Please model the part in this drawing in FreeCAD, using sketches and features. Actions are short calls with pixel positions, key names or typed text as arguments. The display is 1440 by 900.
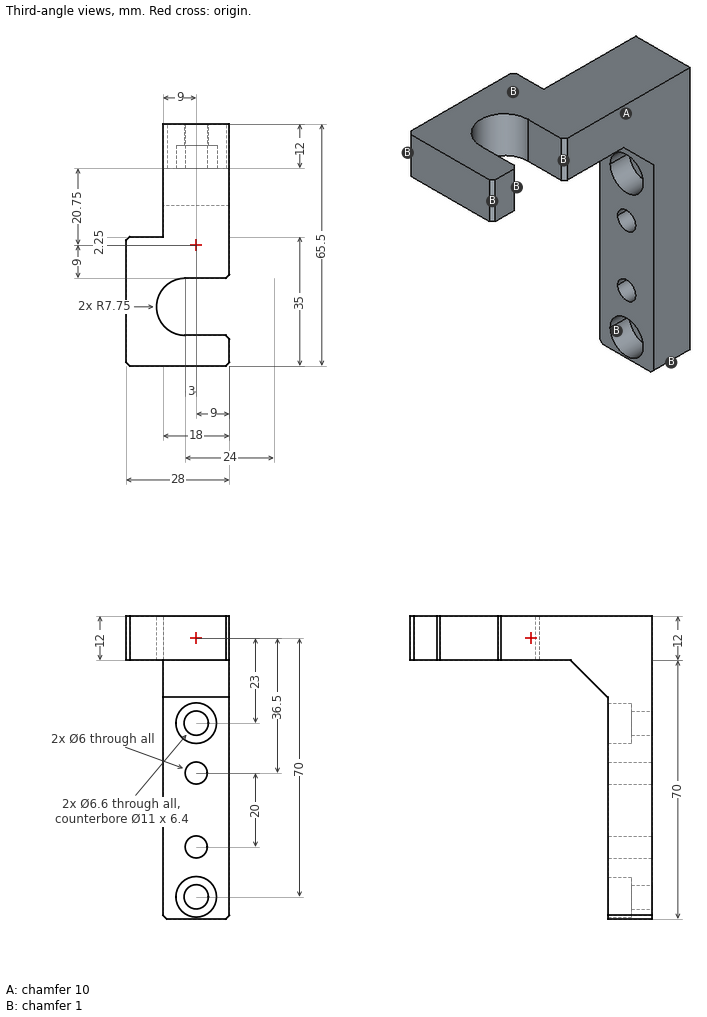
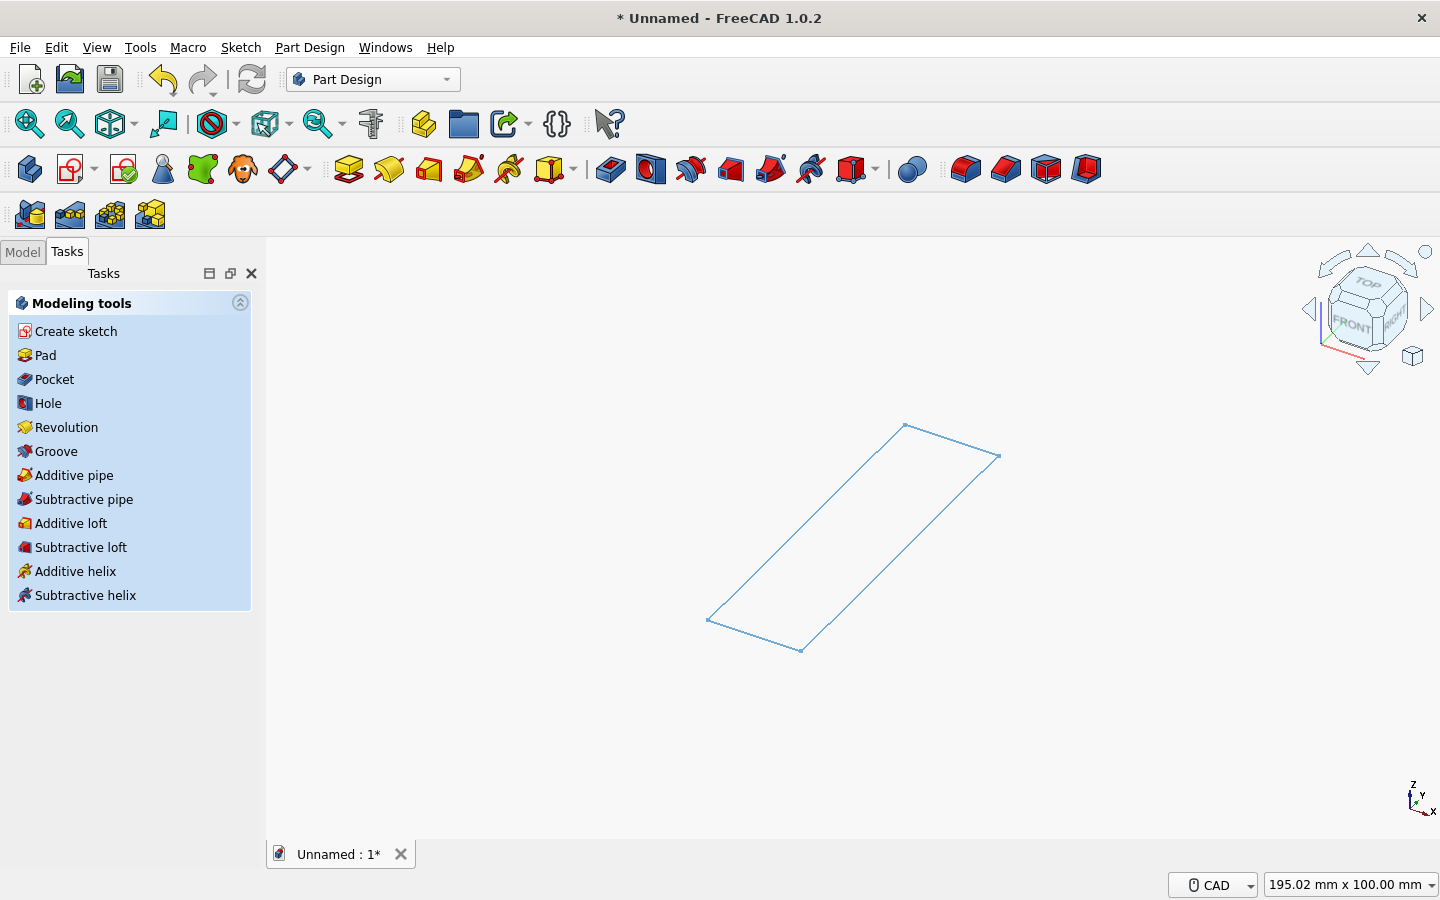
click(350, 170)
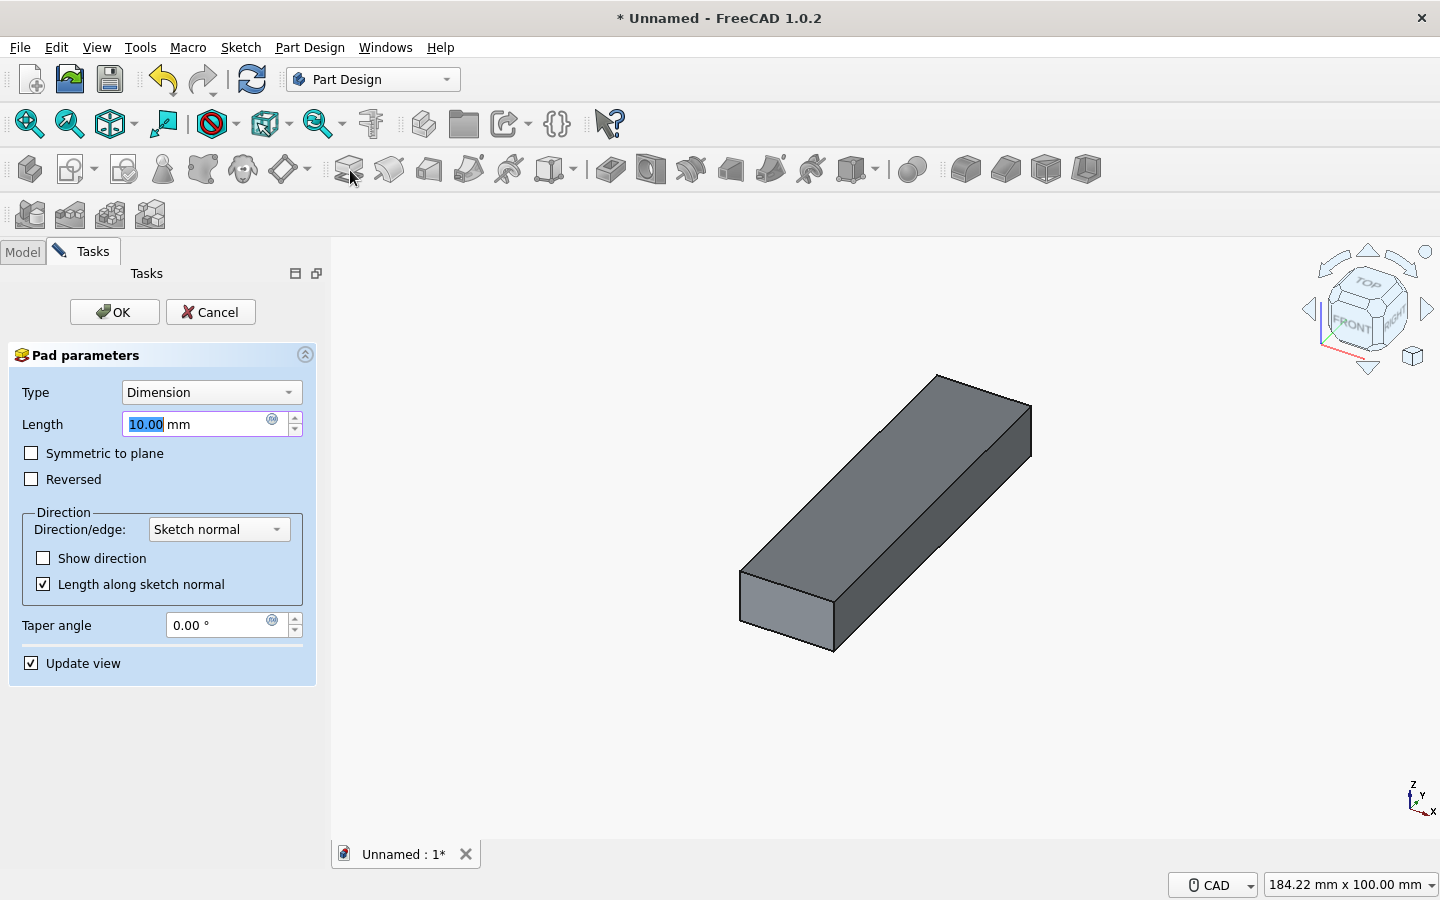
text(12)
key(Tab)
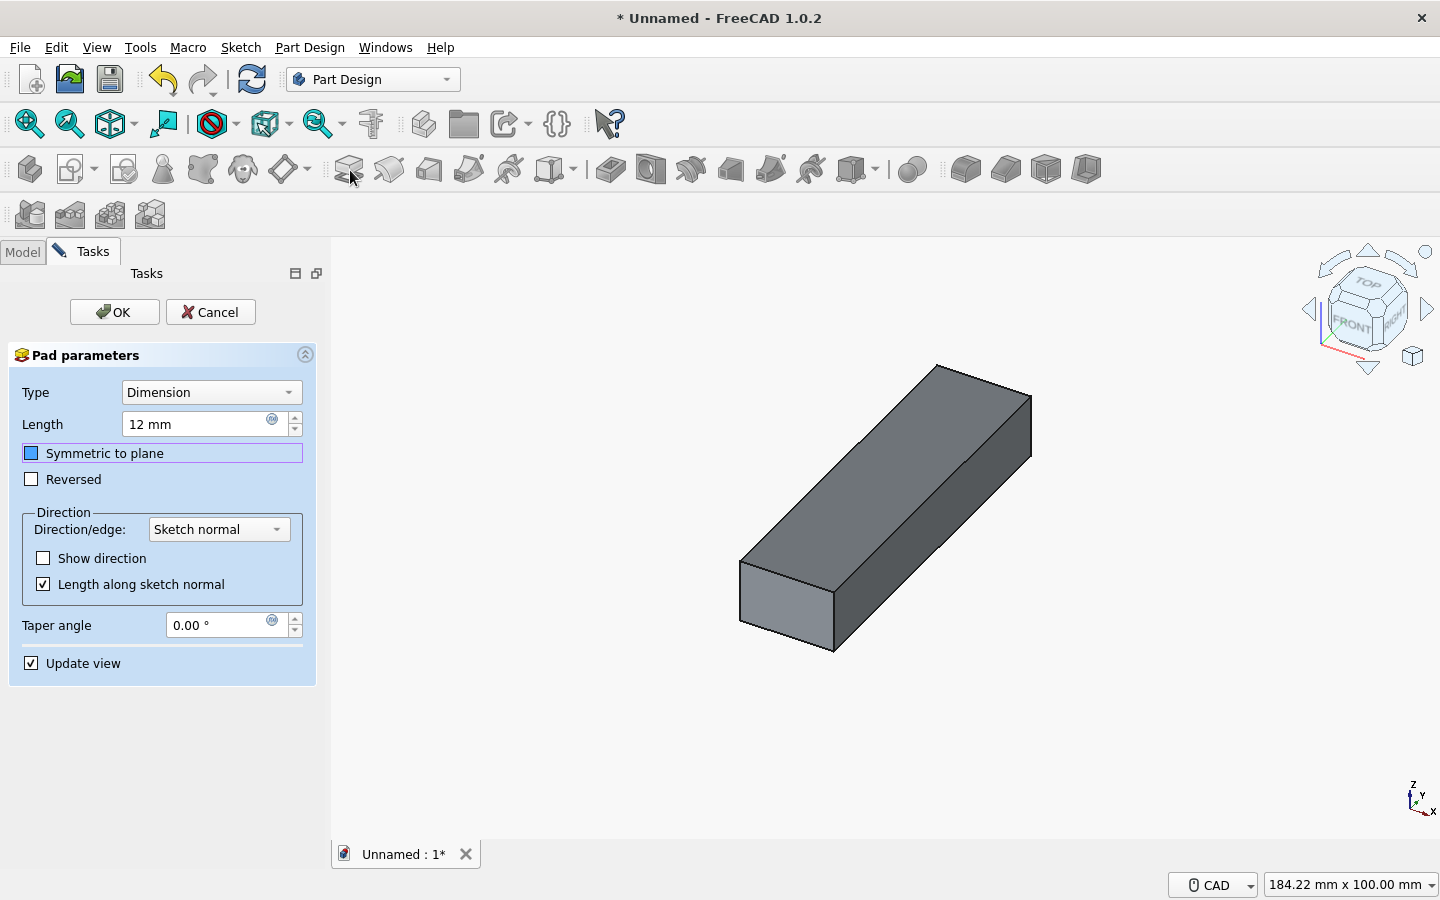
click(30, 453)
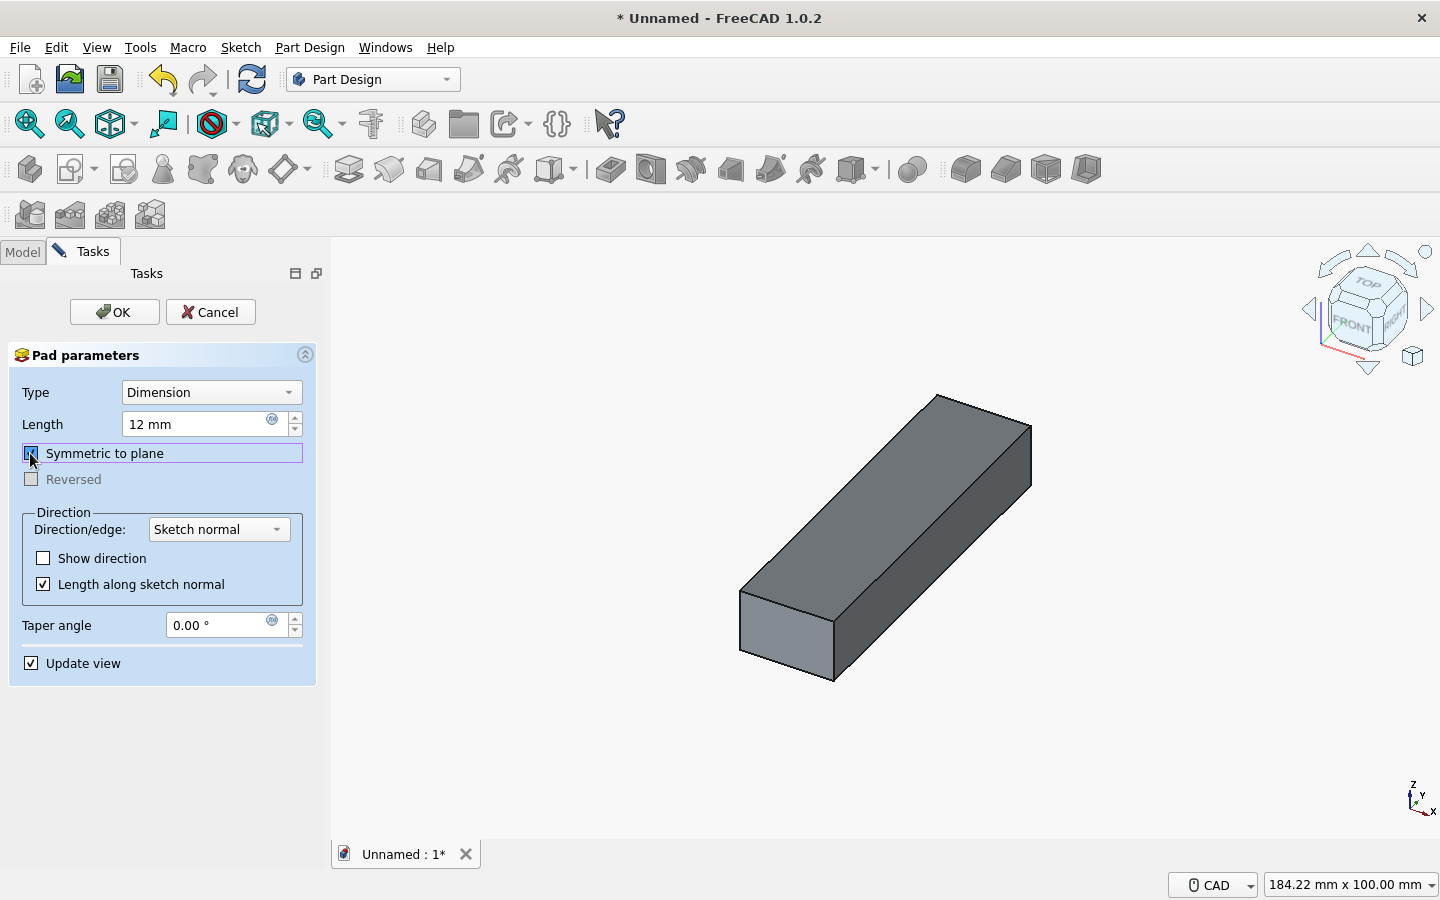
click(115, 312)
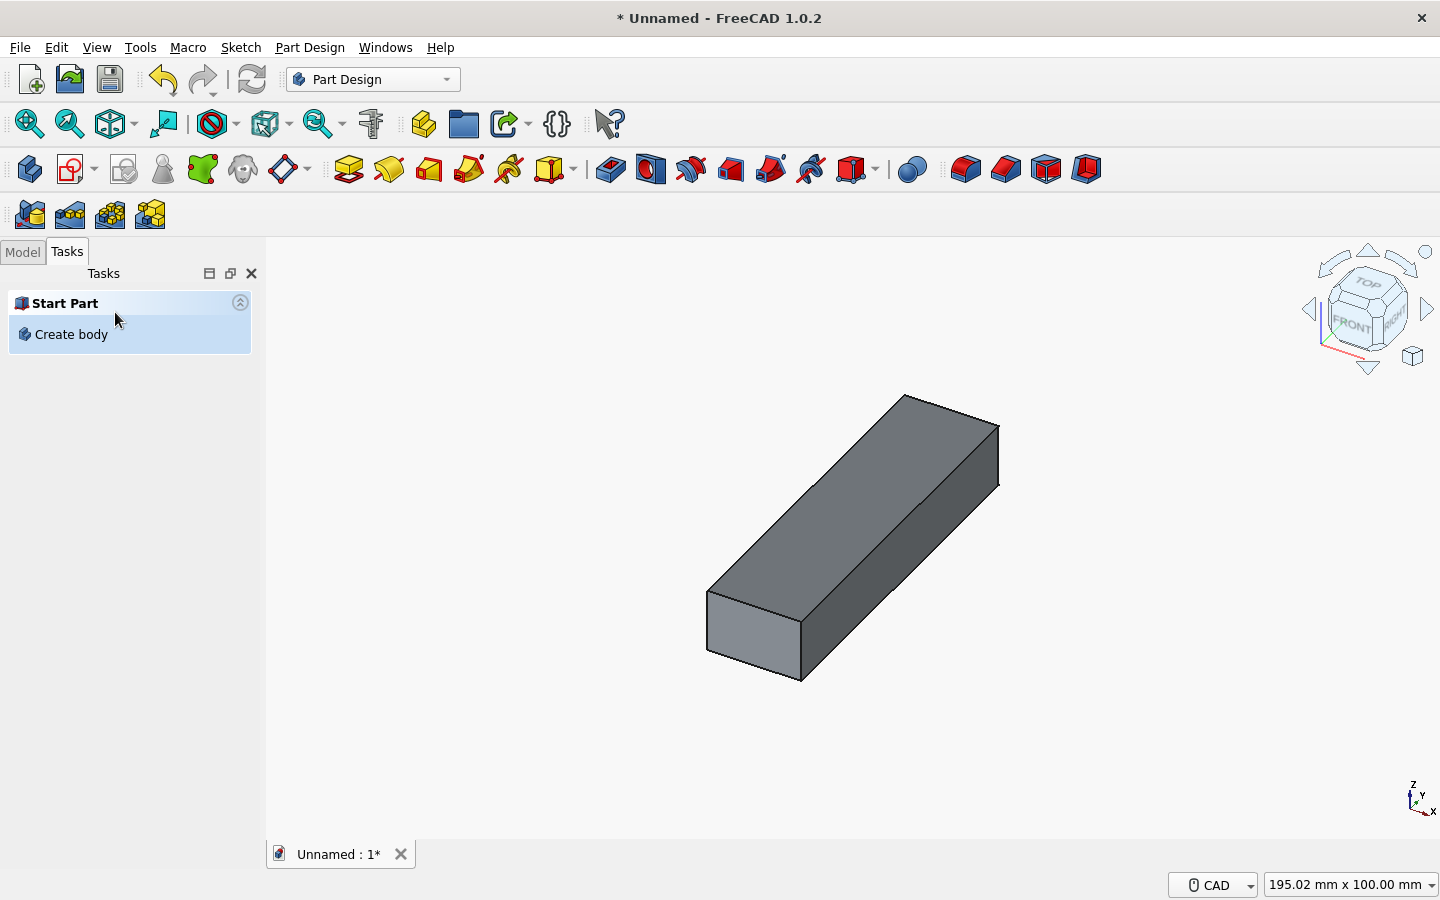
click(909, 451)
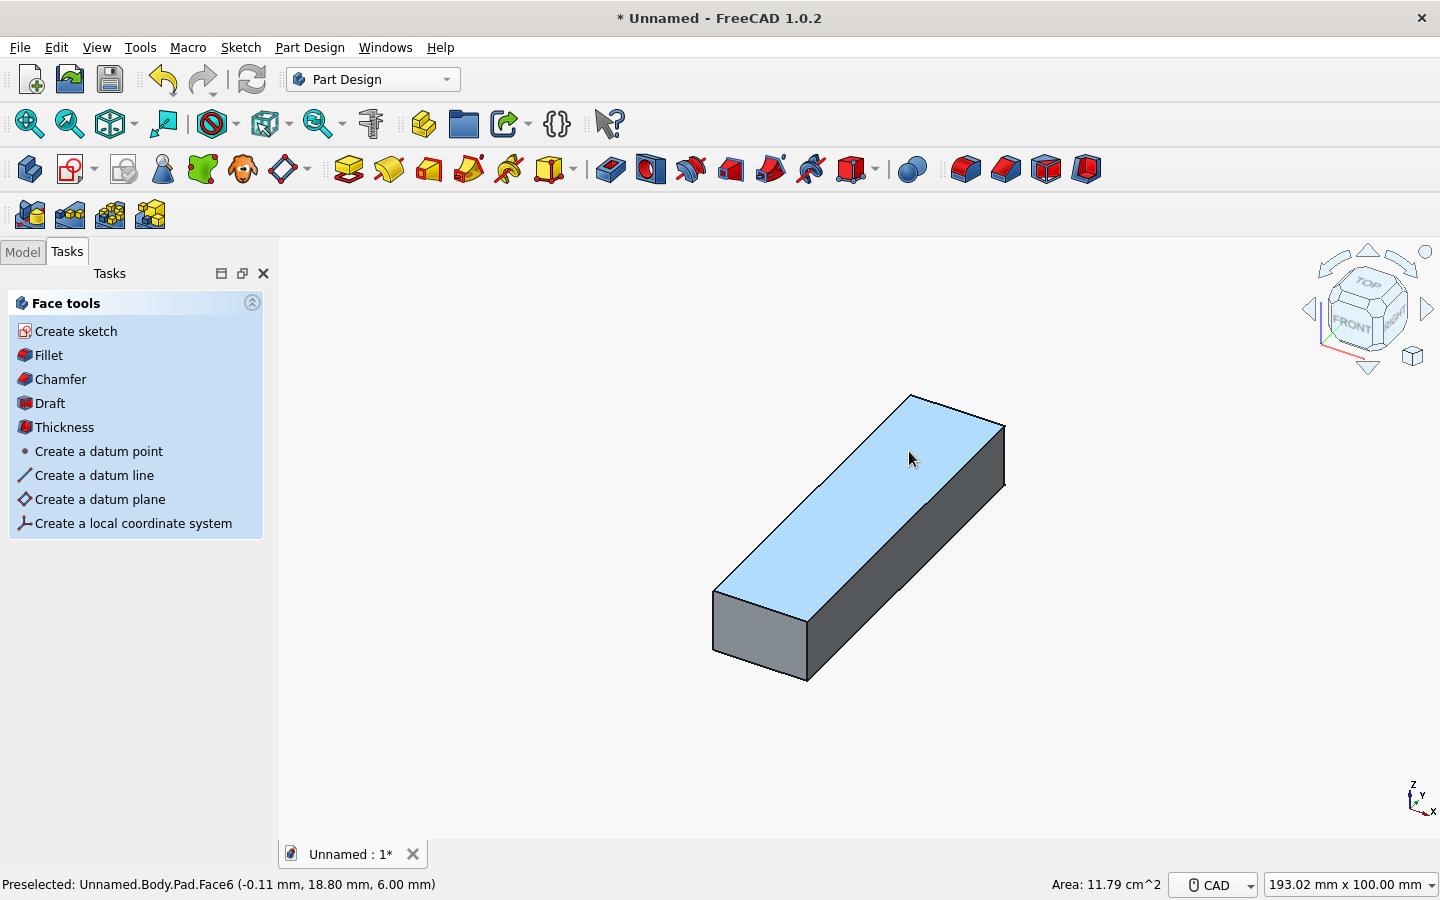
click(70, 170)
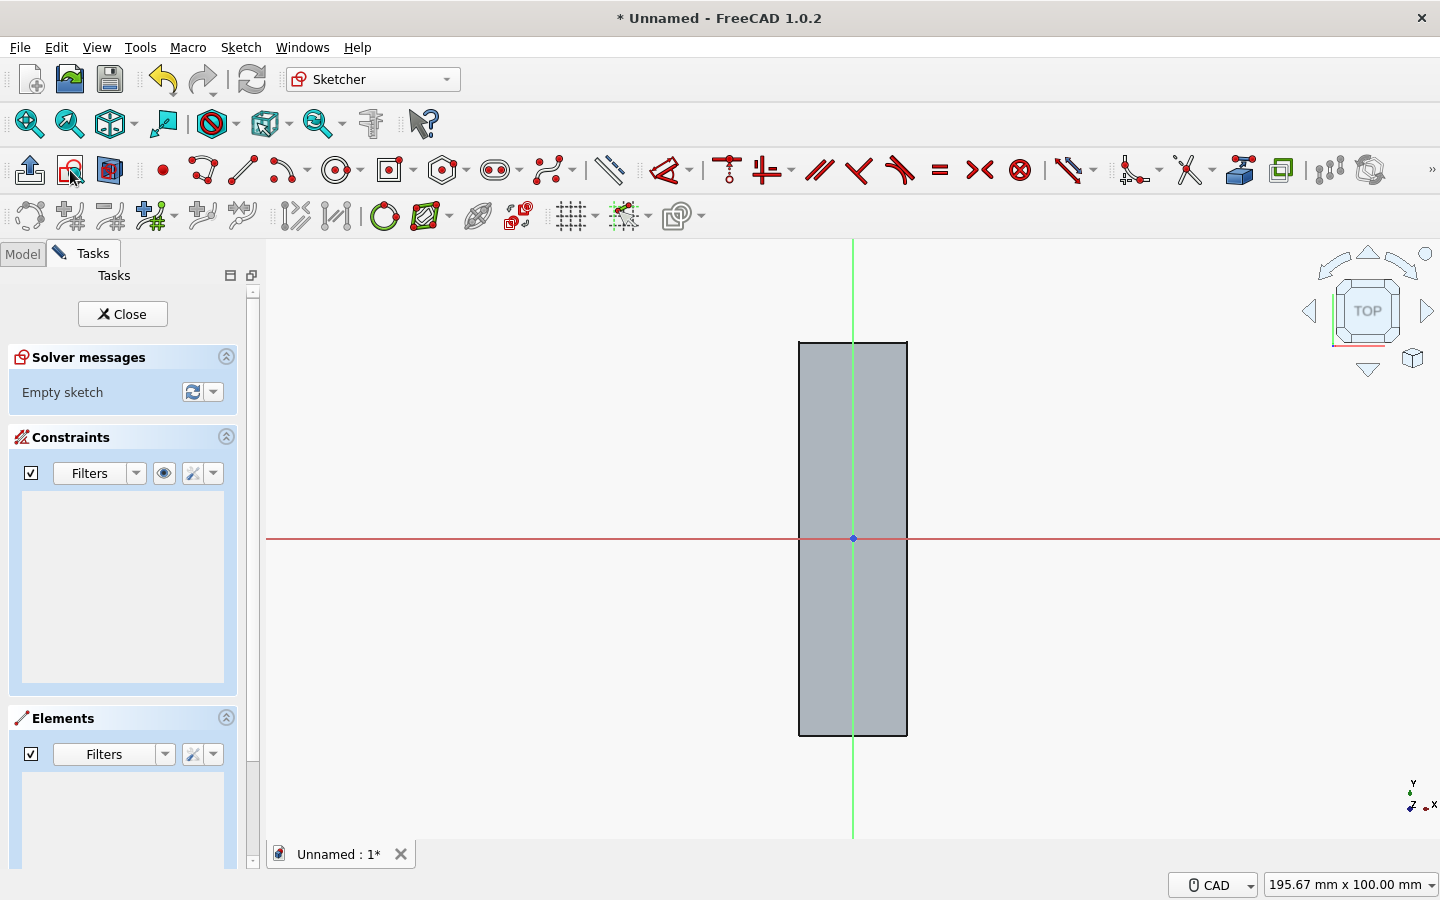
scroll(870, 742, up, 3)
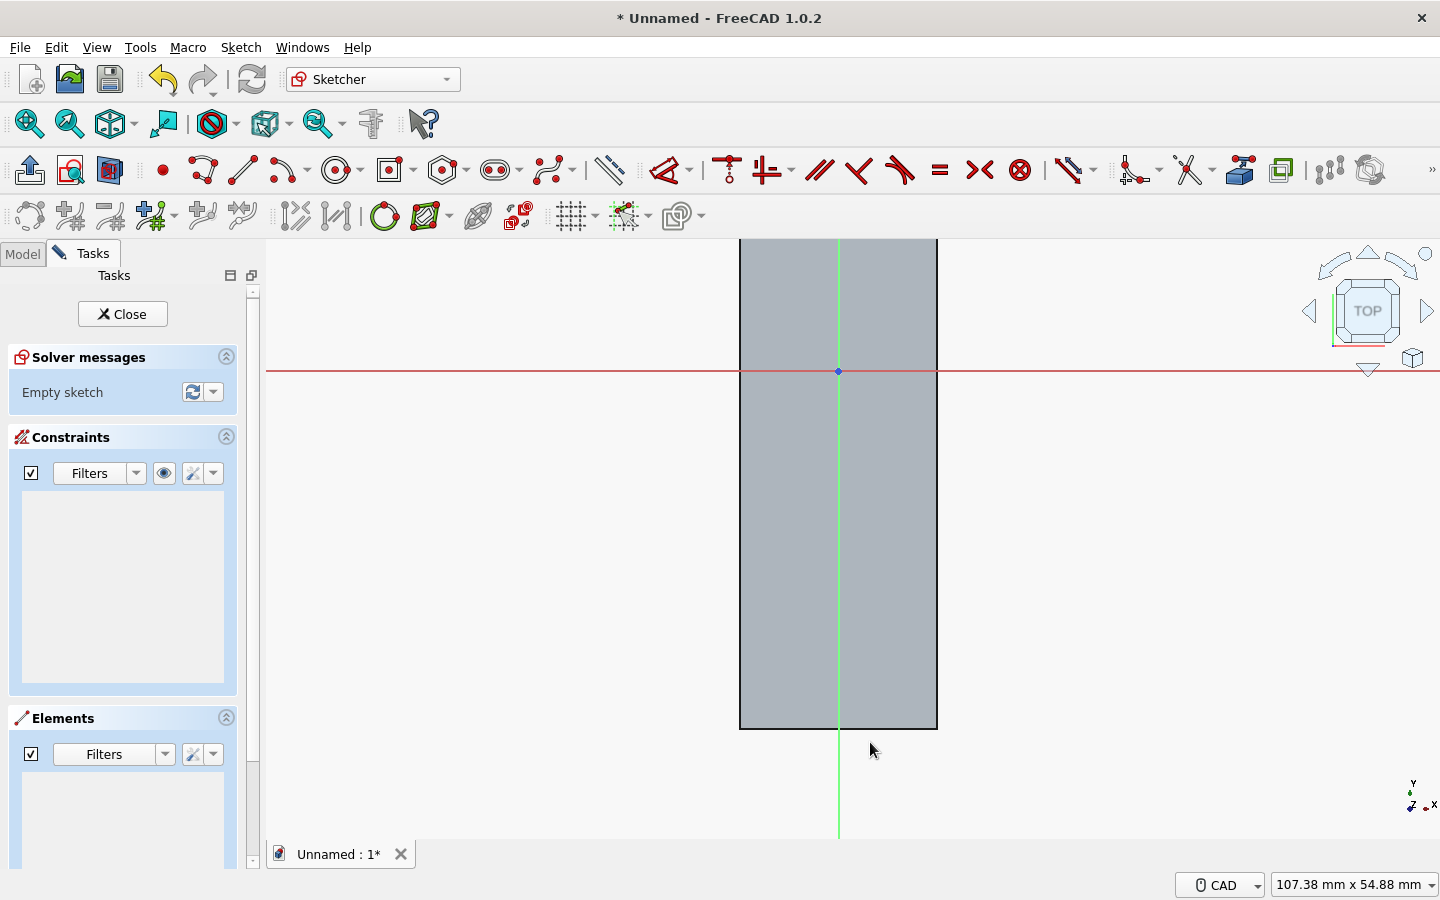
click(416, 170)